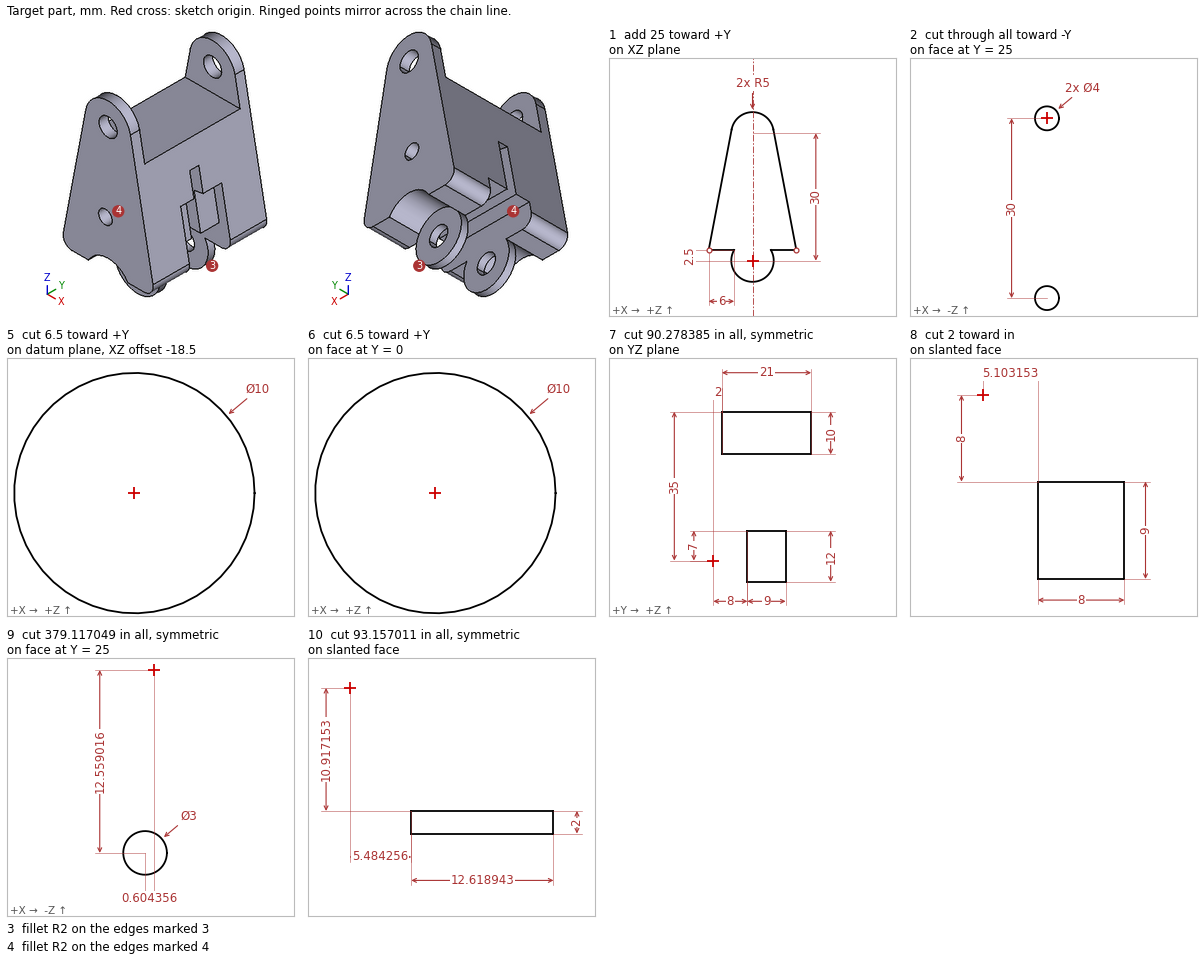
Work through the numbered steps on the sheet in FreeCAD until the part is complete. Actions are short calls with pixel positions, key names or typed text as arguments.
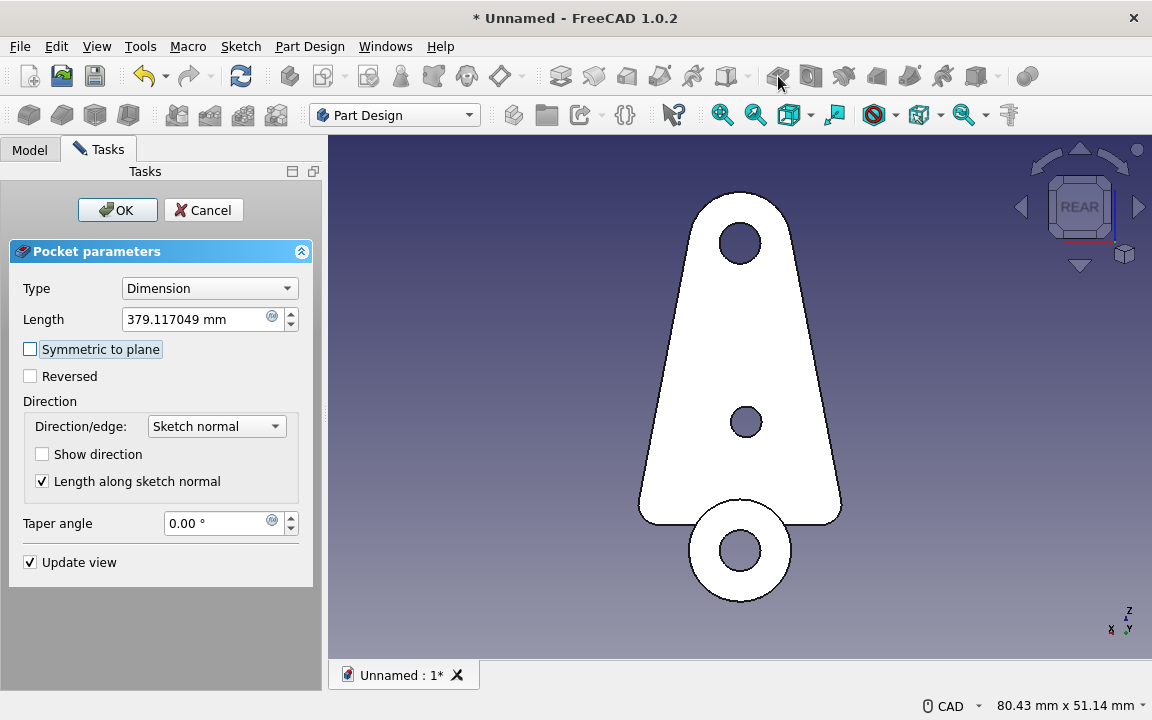
click(31, 349)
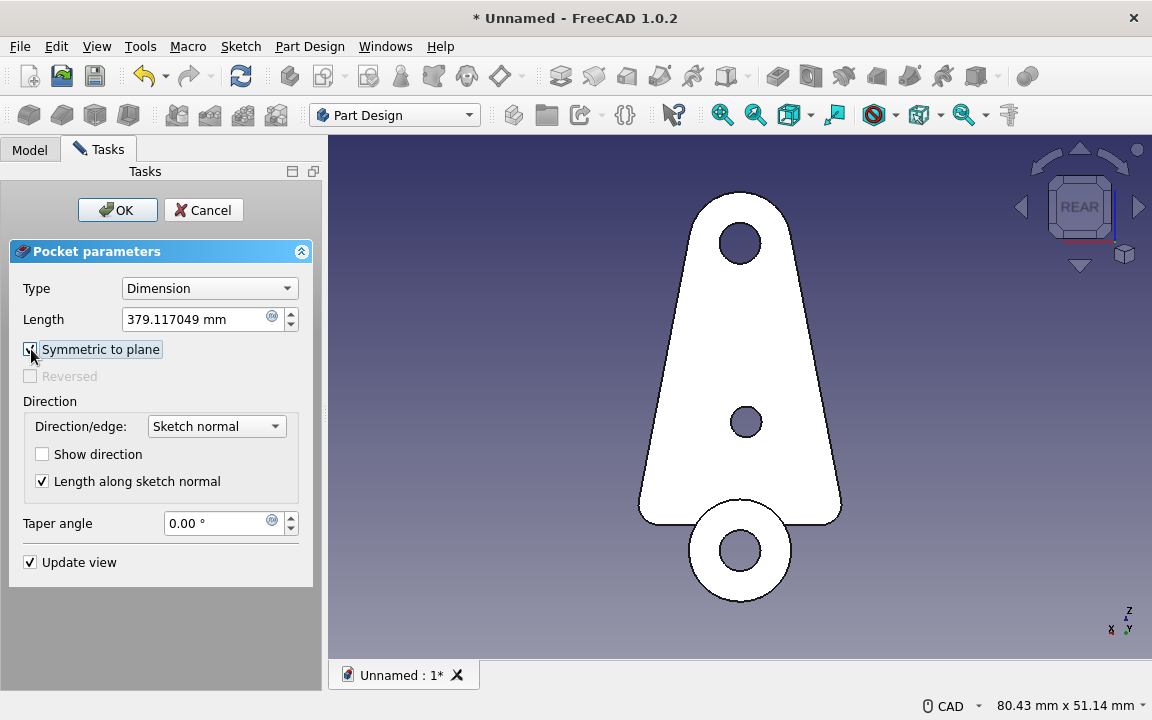
click(118, 210)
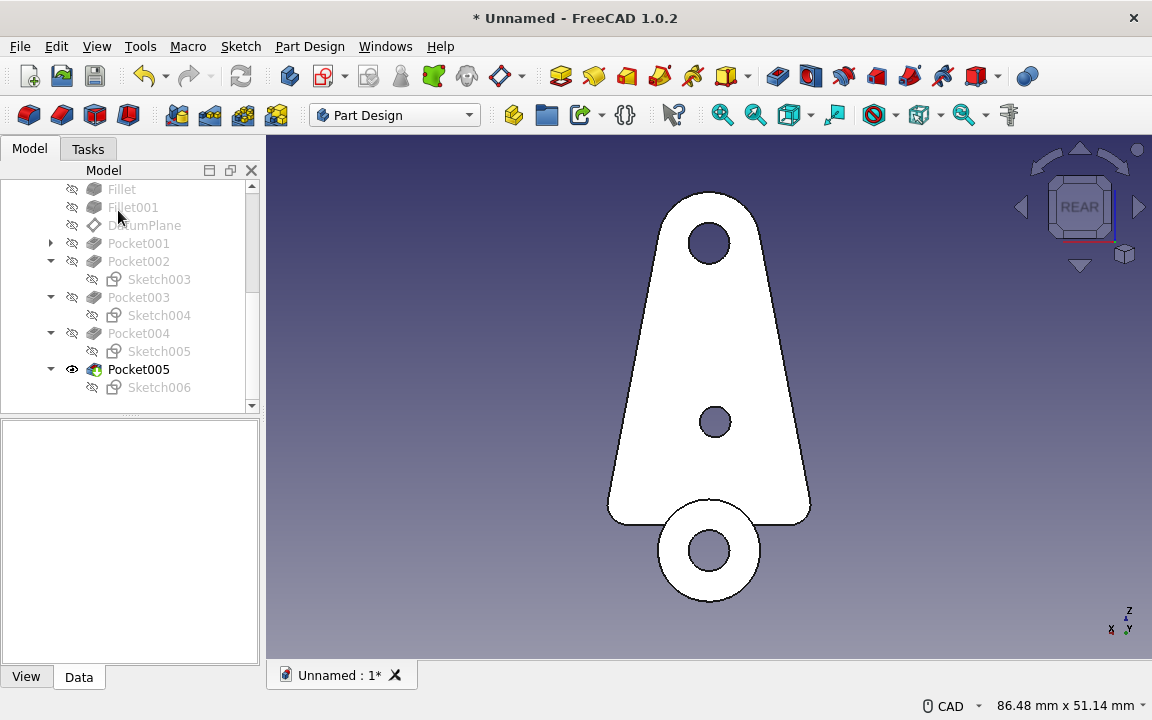
key(0)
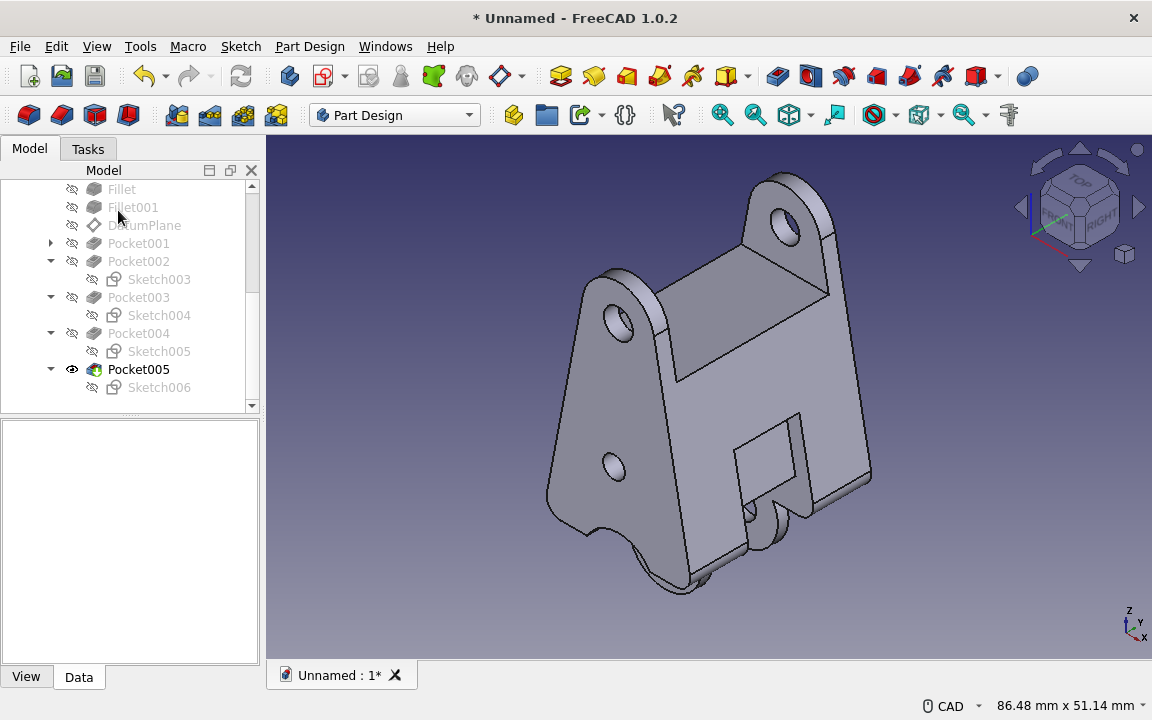
click(758, 460)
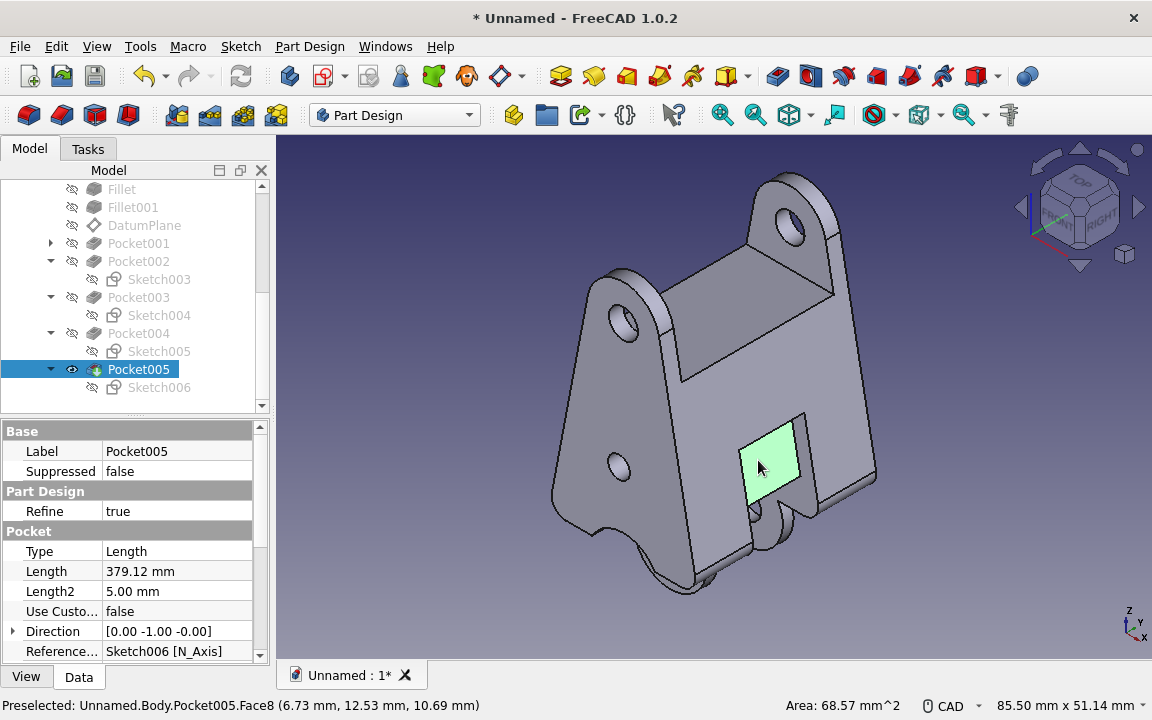
click(322, 76)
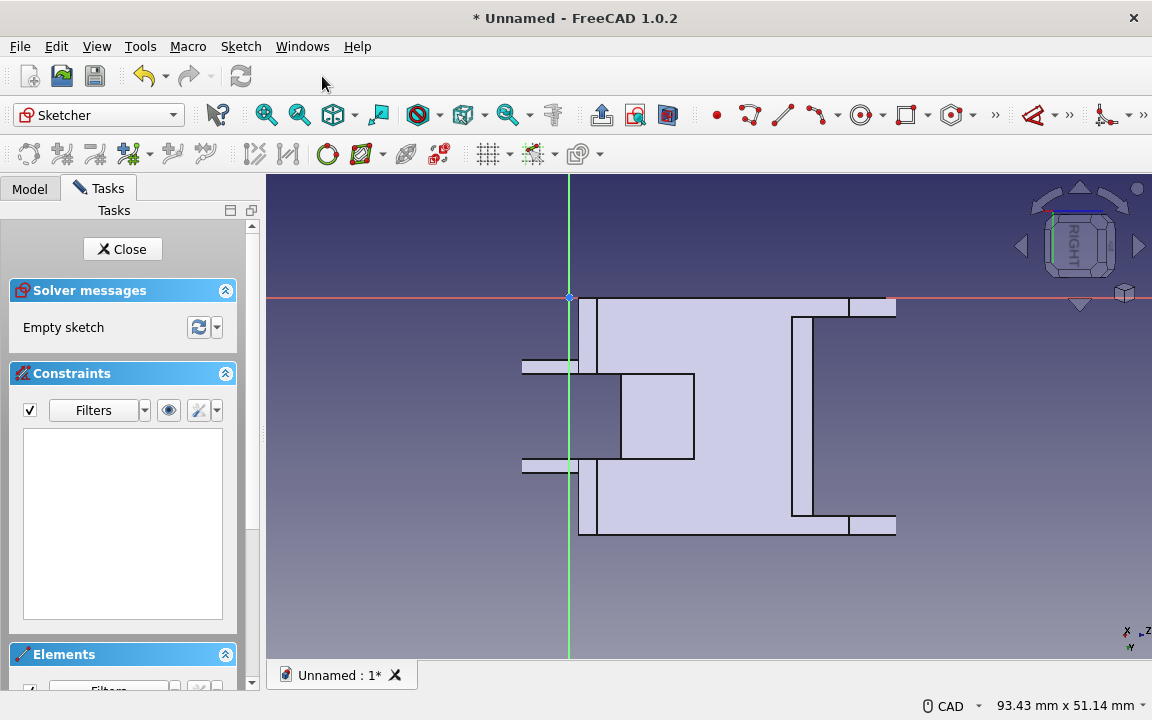
key(q)
key(s)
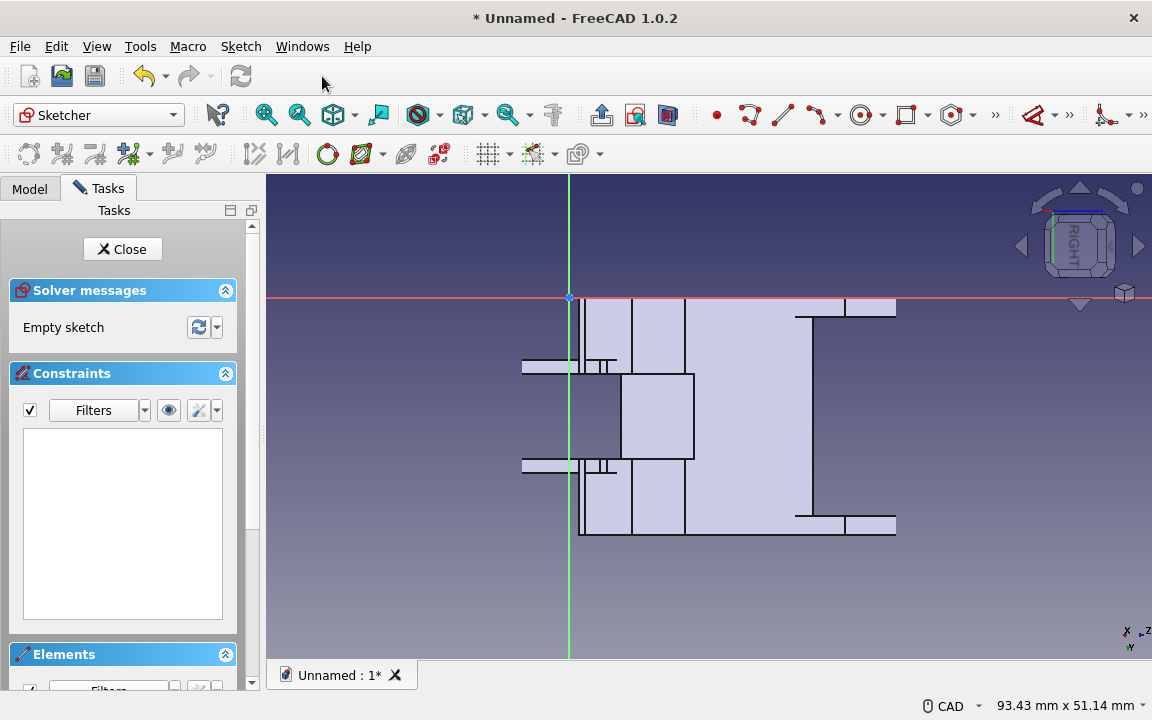
scroll(664, 326, up, 5)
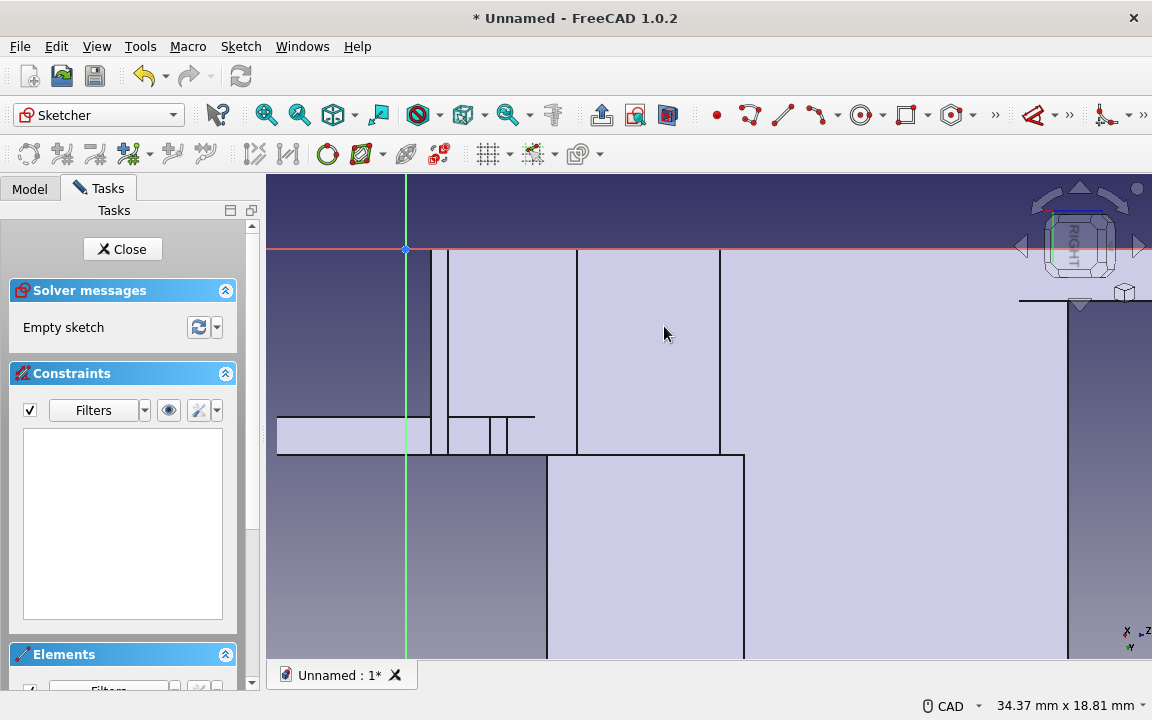
key(g)
key(r)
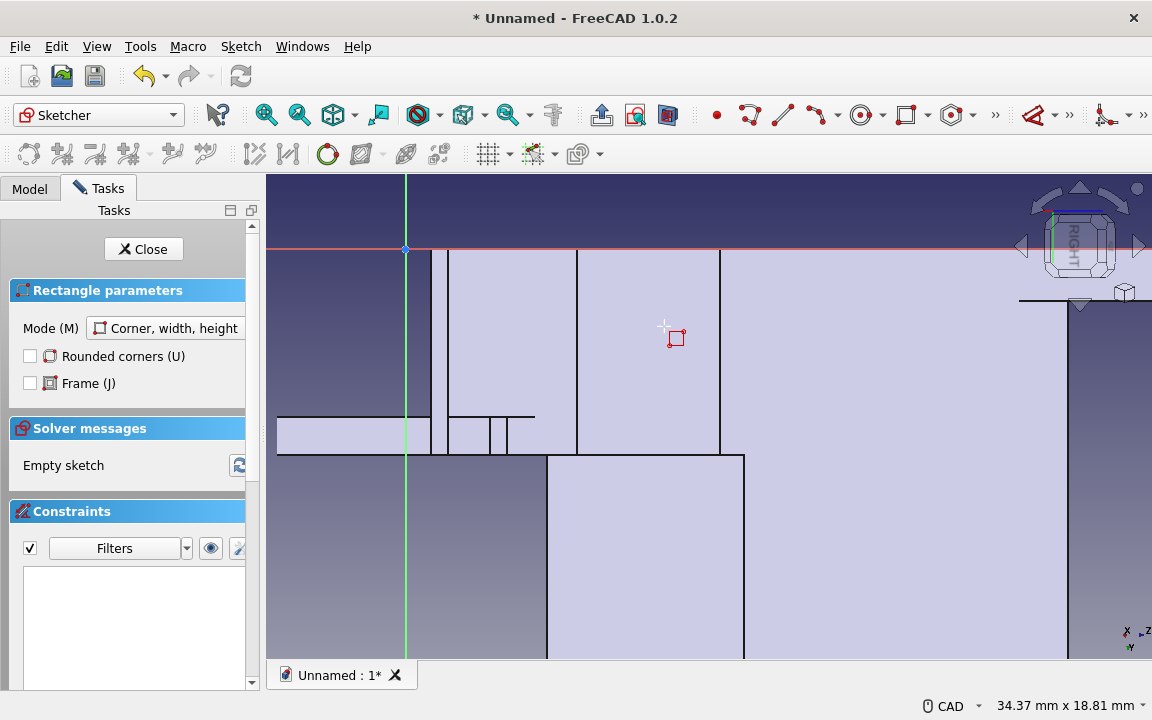
click(547, 531)
move(873, 582)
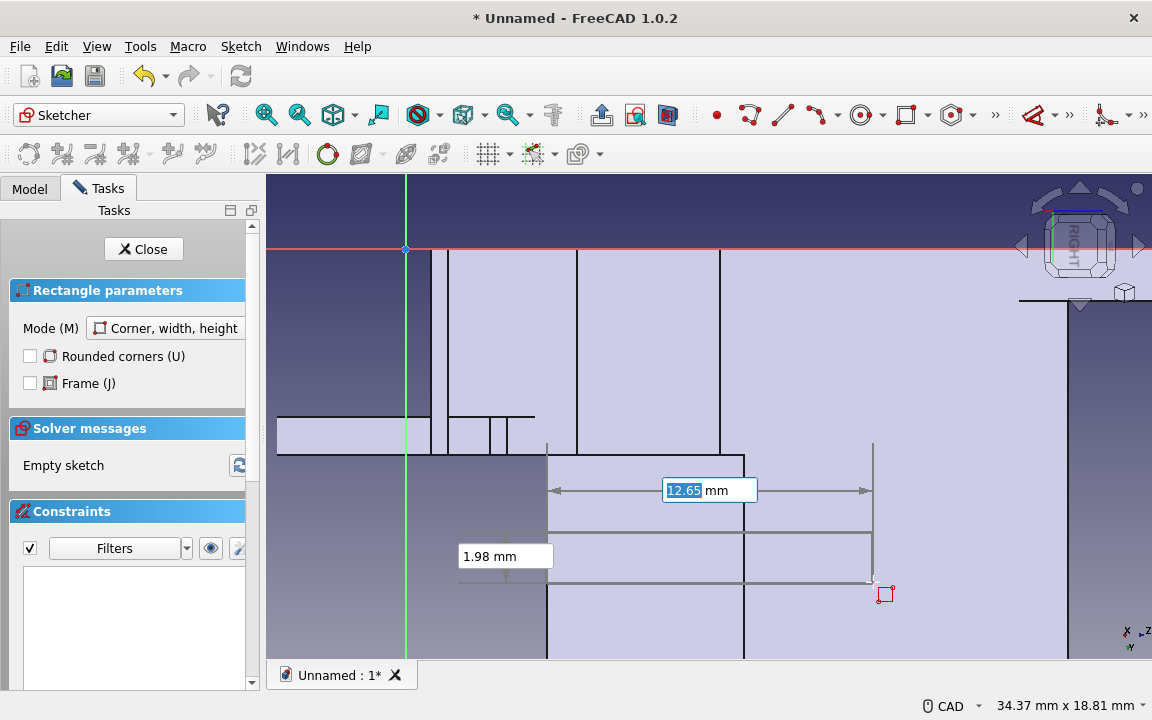
text(12.618943)
key(Tab)
text(2)
key(Return)
key(Escape)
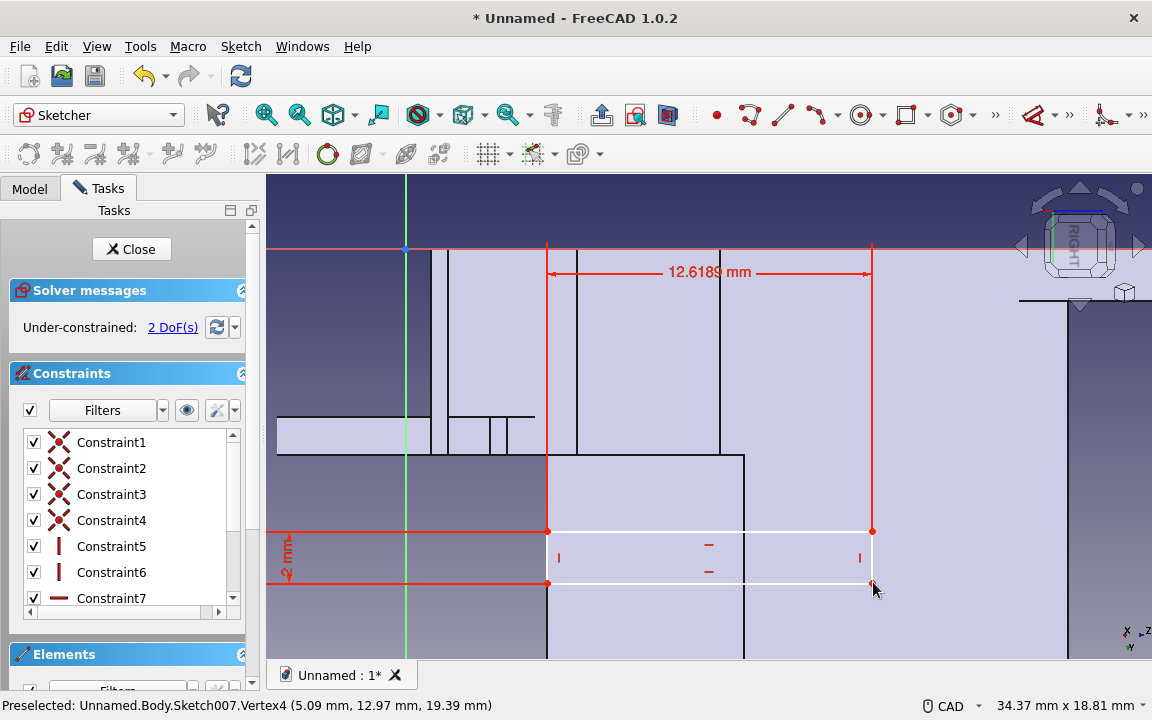
click(1032, 116)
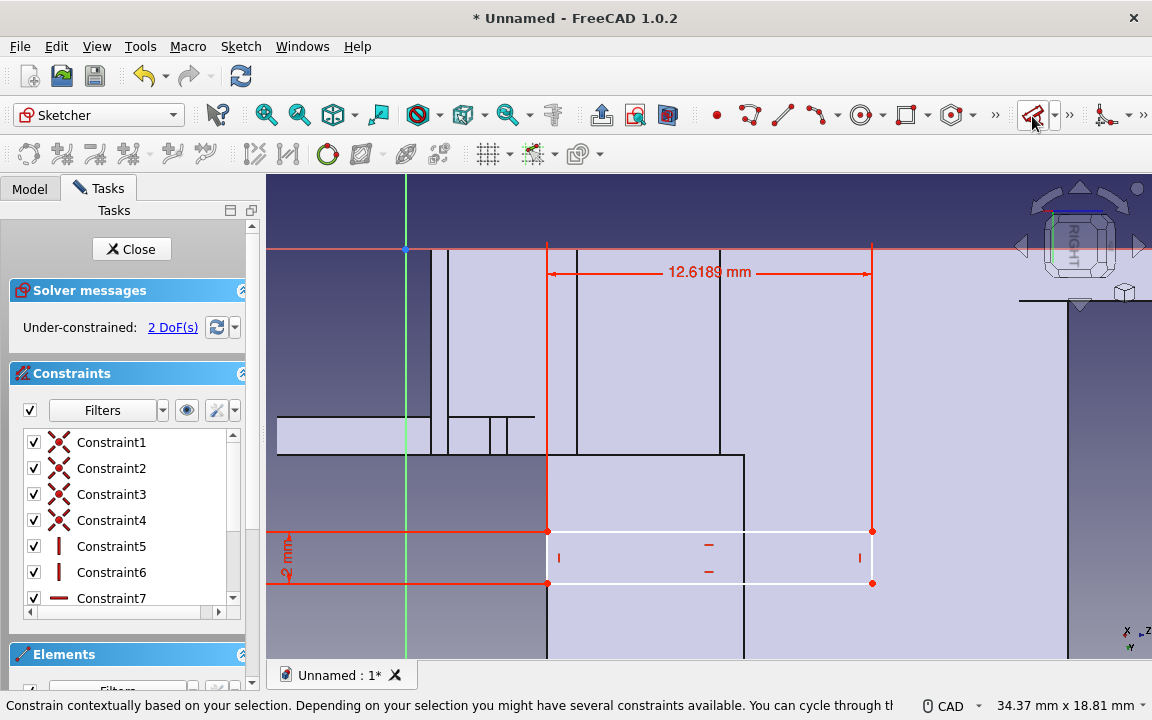
click(547, 532)
click(476, 215)